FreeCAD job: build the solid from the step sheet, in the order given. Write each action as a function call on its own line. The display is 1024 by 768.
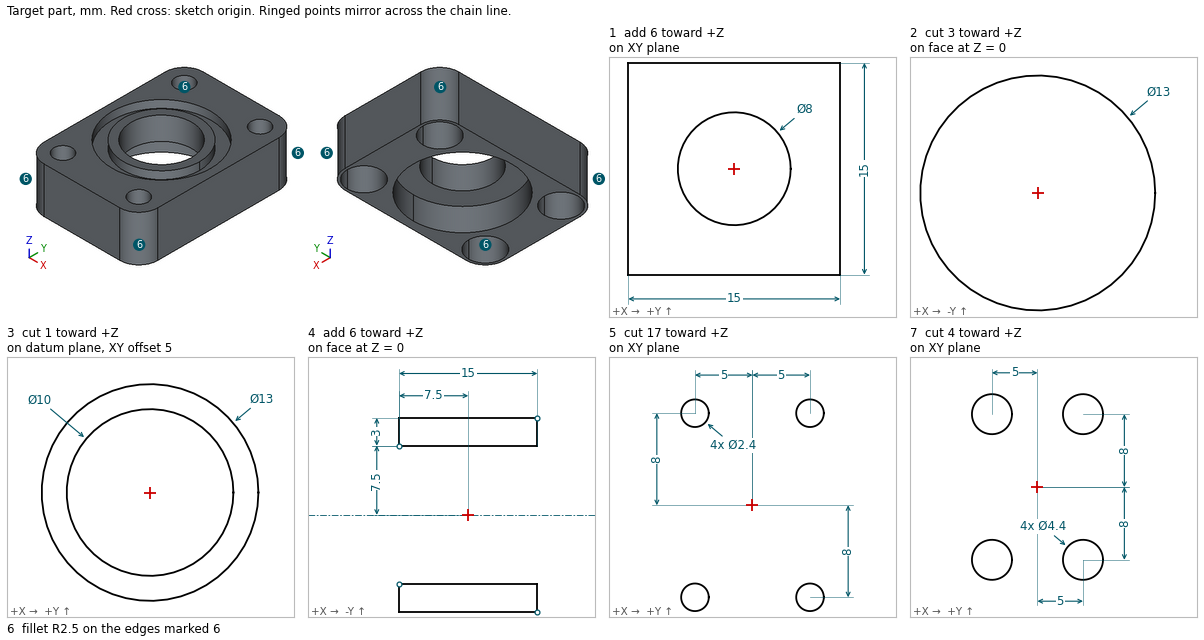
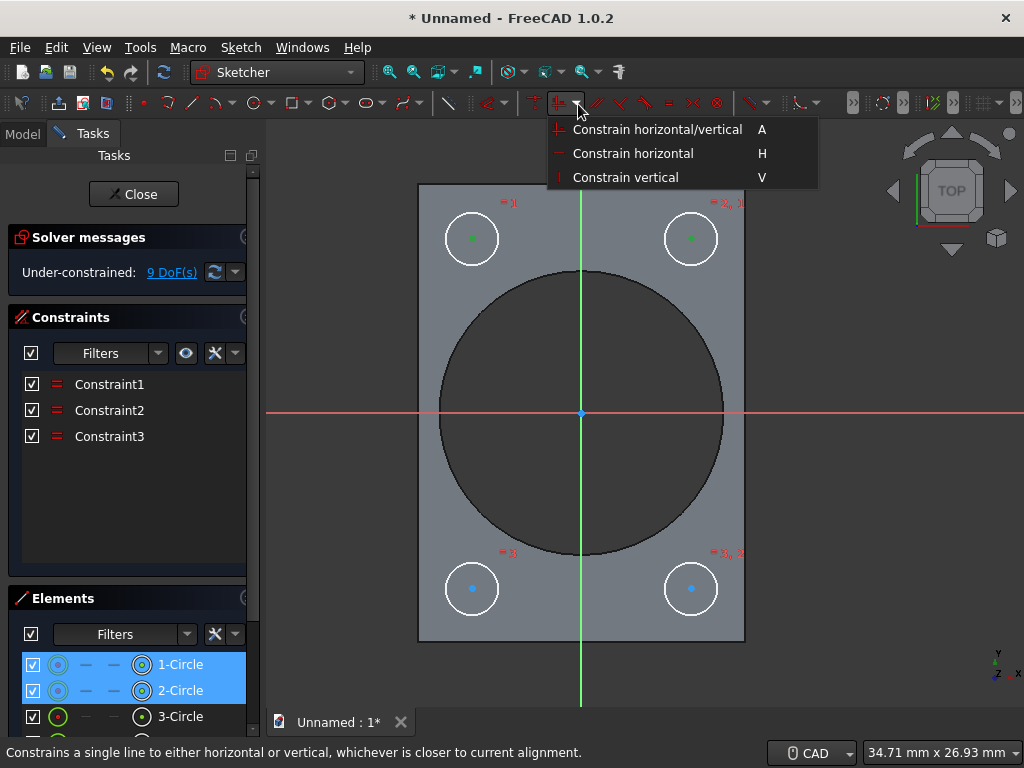
click(683, 153)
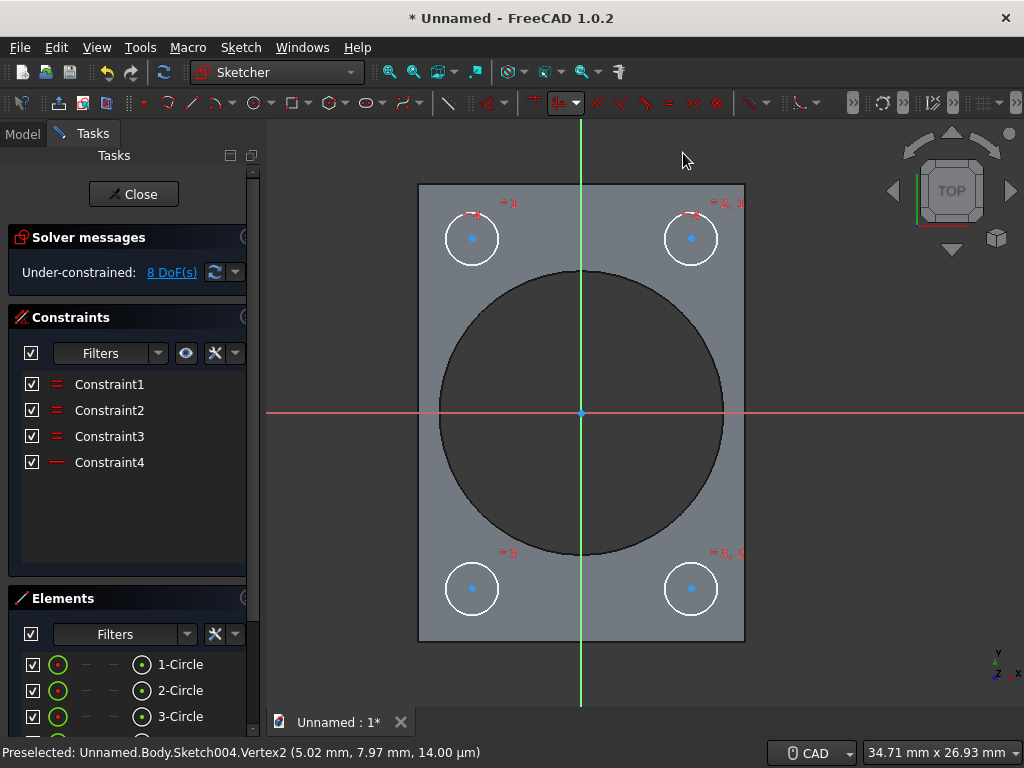
click(691, 239)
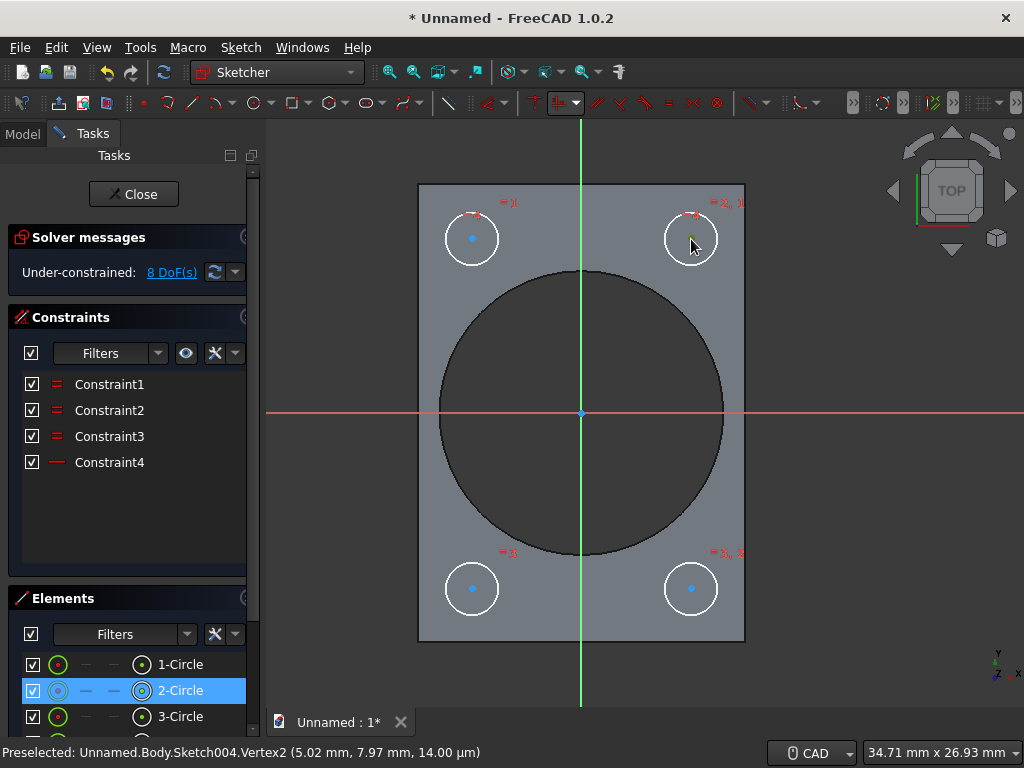
click(691, 589)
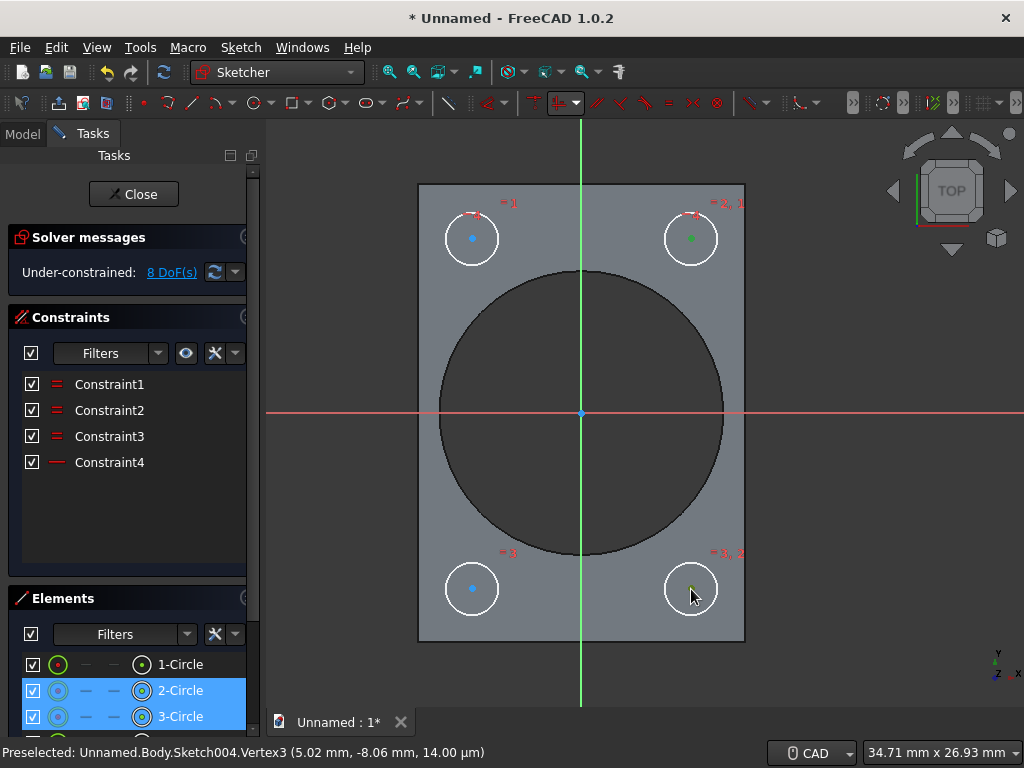
click(578, 104)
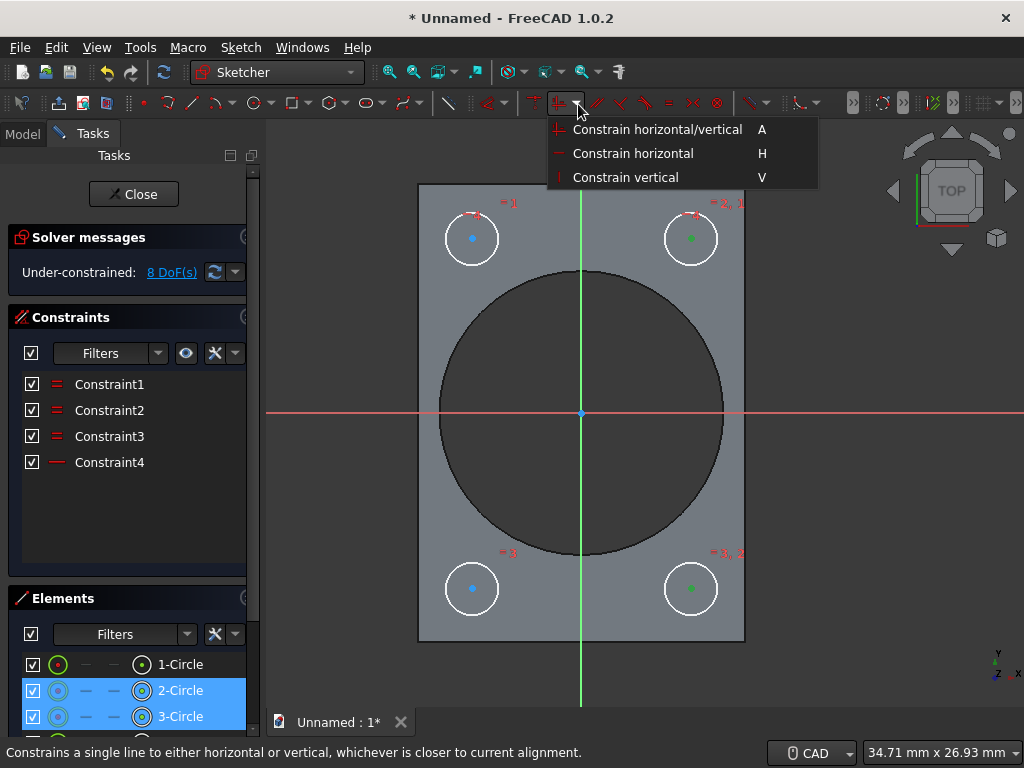
click(683, 177)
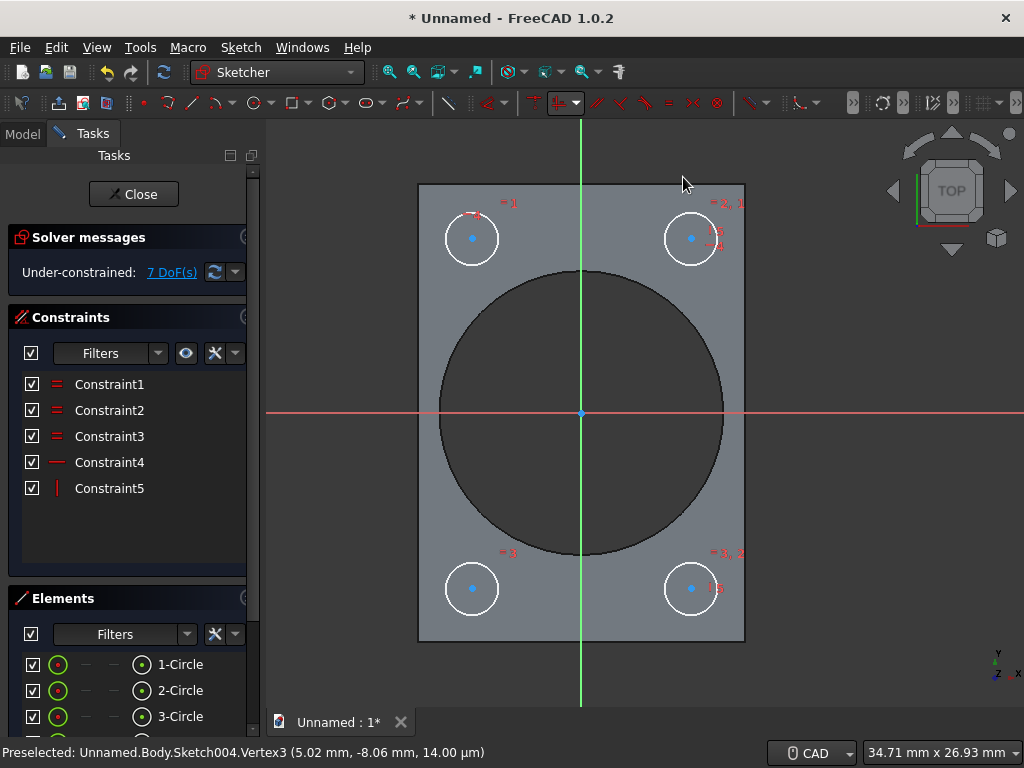
click(472, 239)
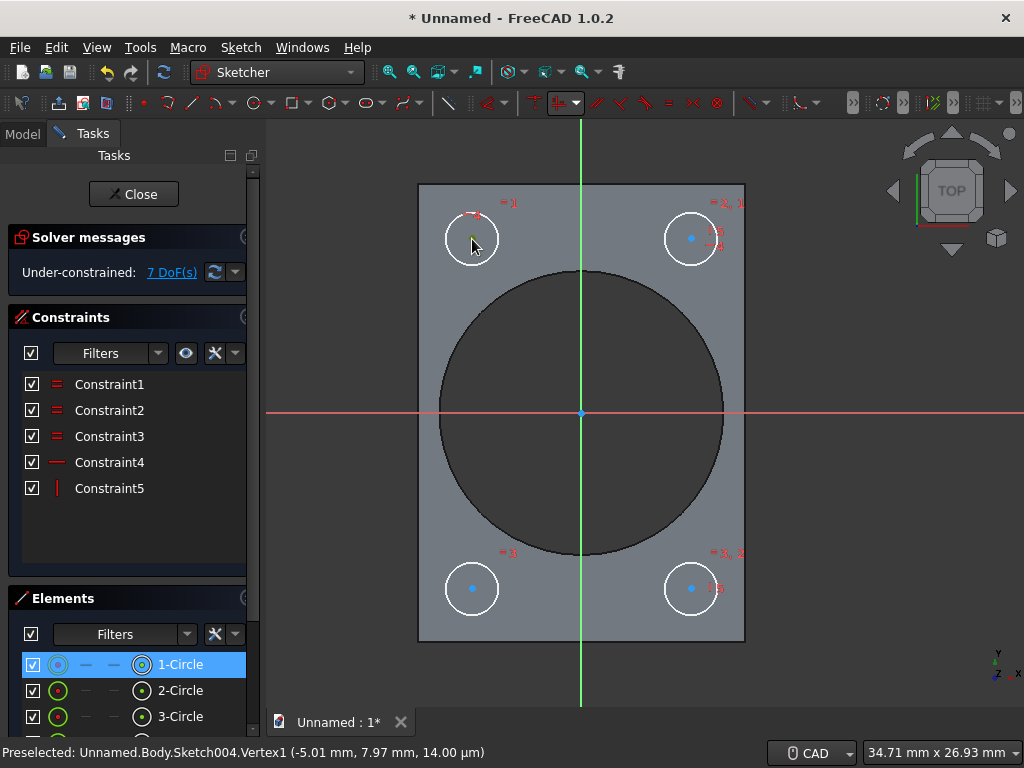
click(472, 589)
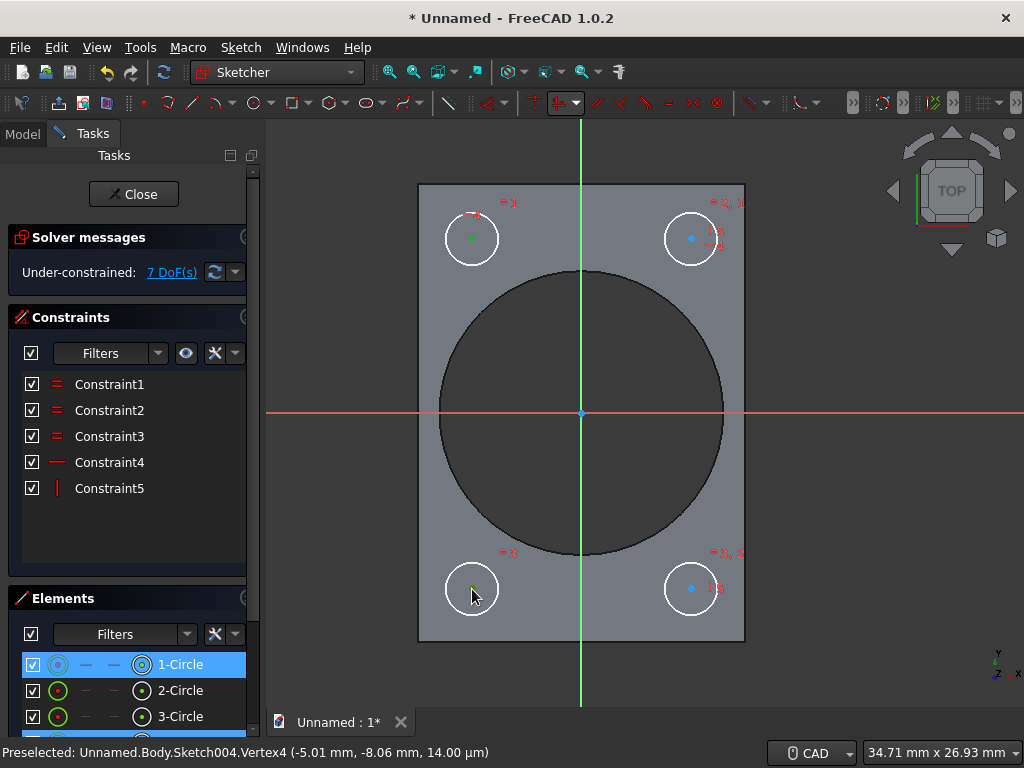
key(v)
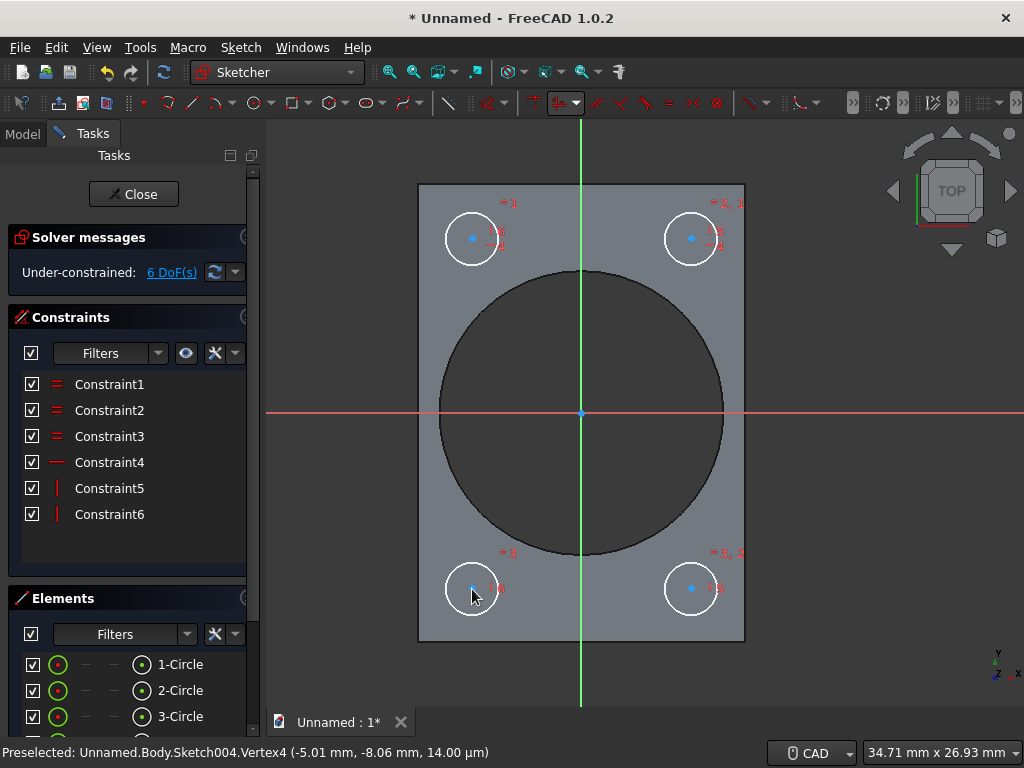
click(691, 589)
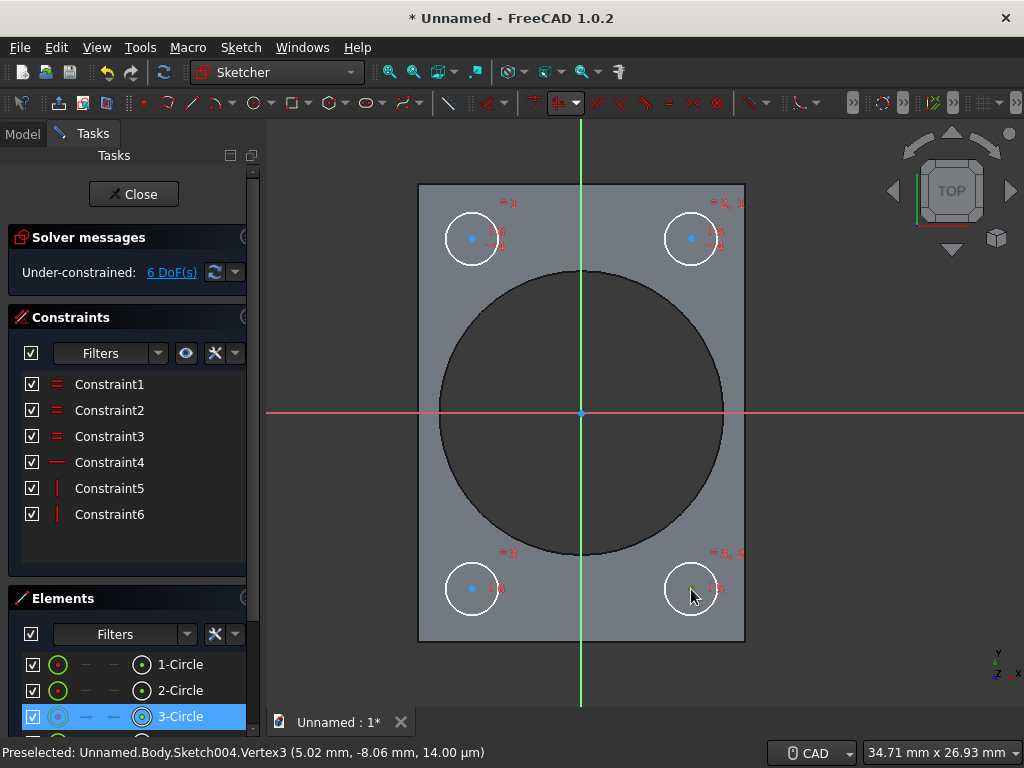
click(472, 589)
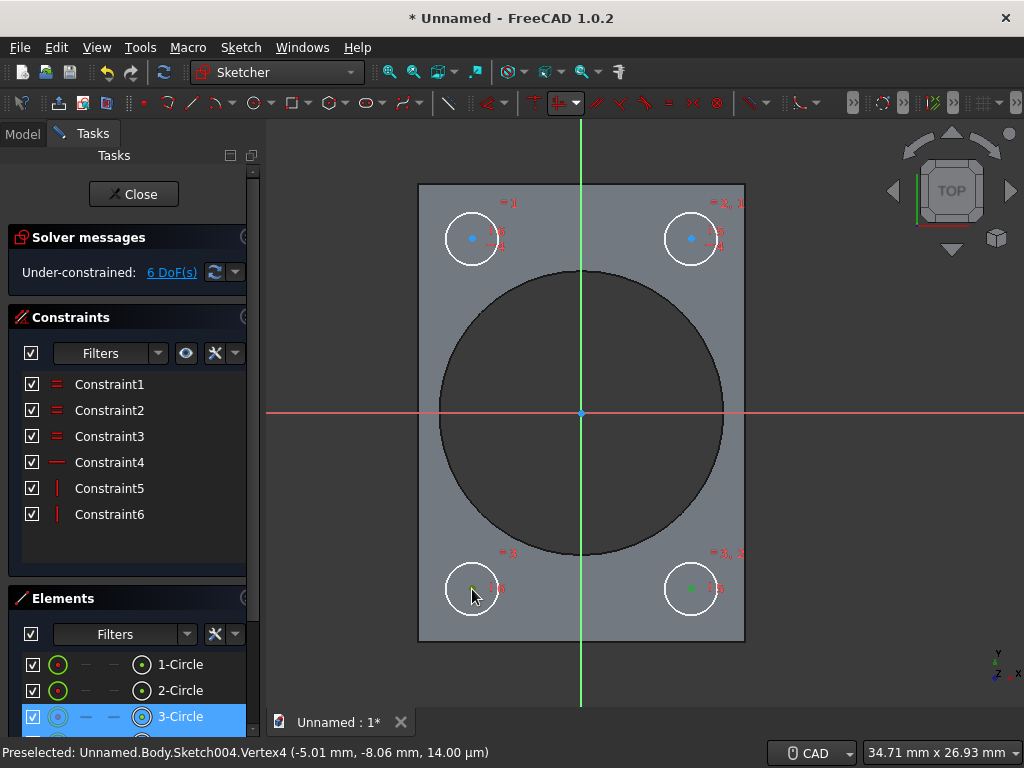
click(578, 104)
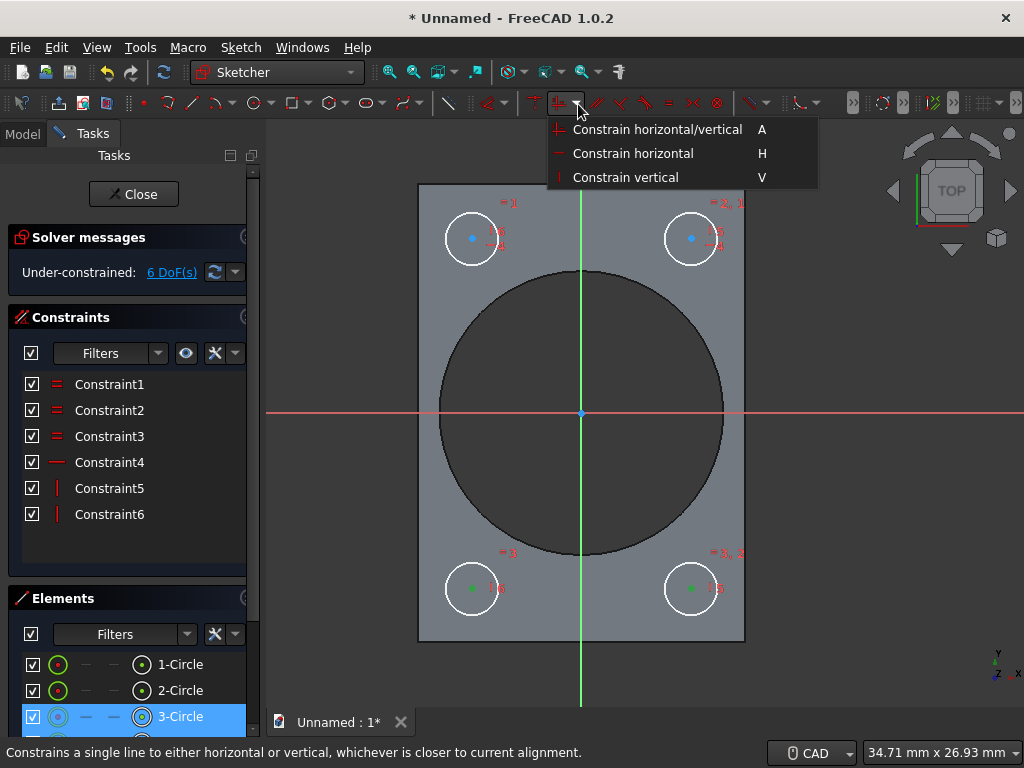
click(683, 153)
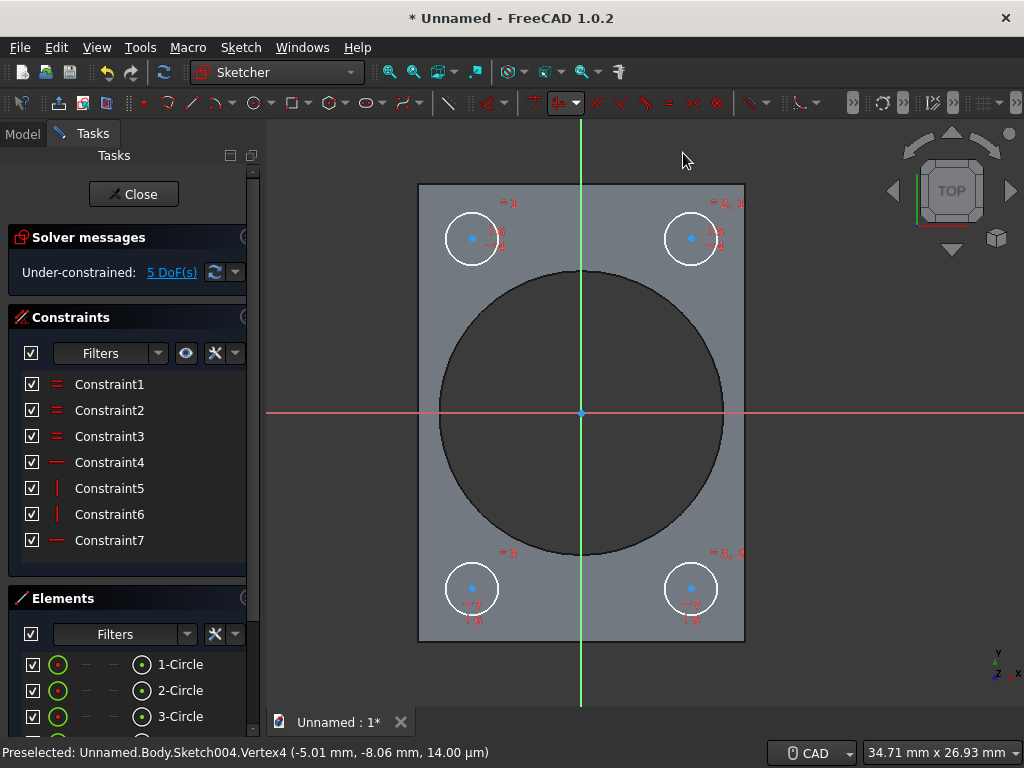
click(488, 104)